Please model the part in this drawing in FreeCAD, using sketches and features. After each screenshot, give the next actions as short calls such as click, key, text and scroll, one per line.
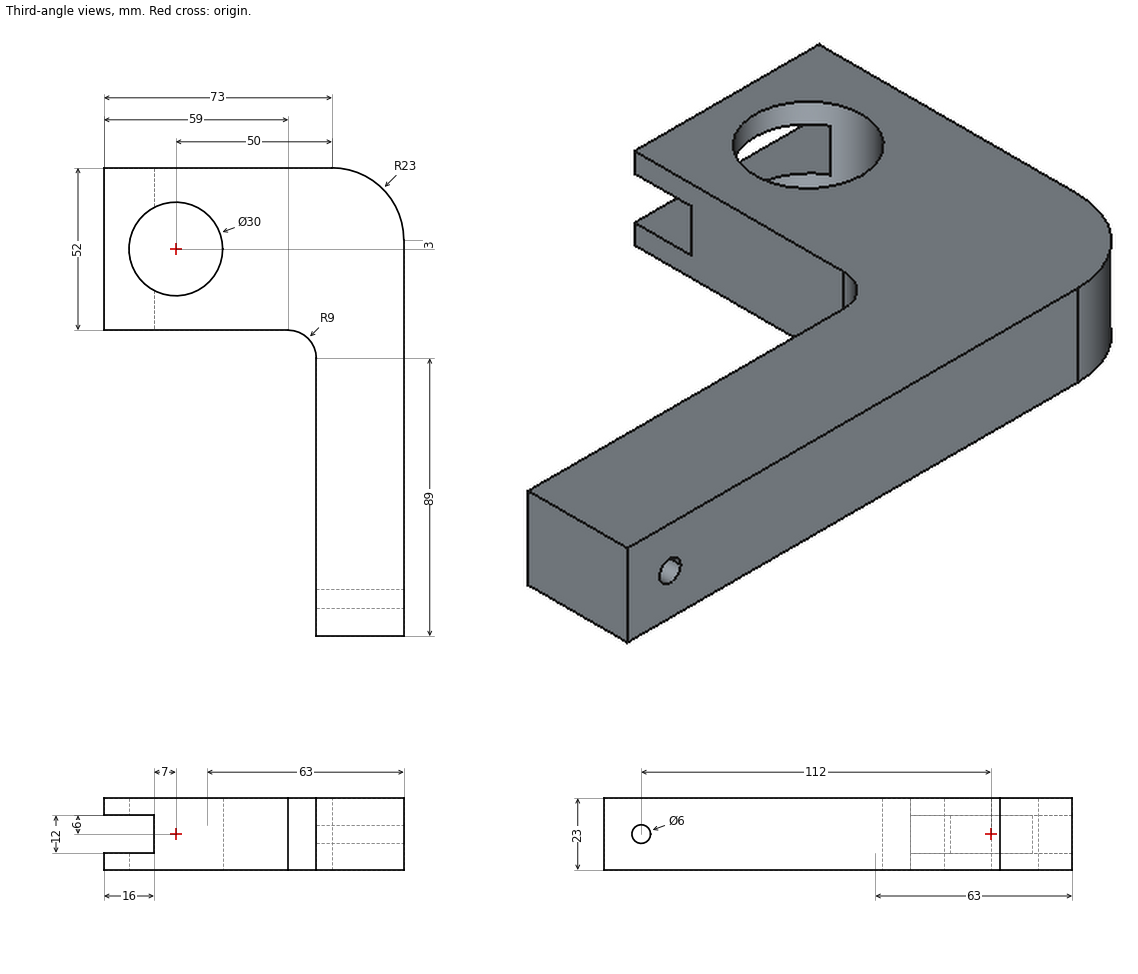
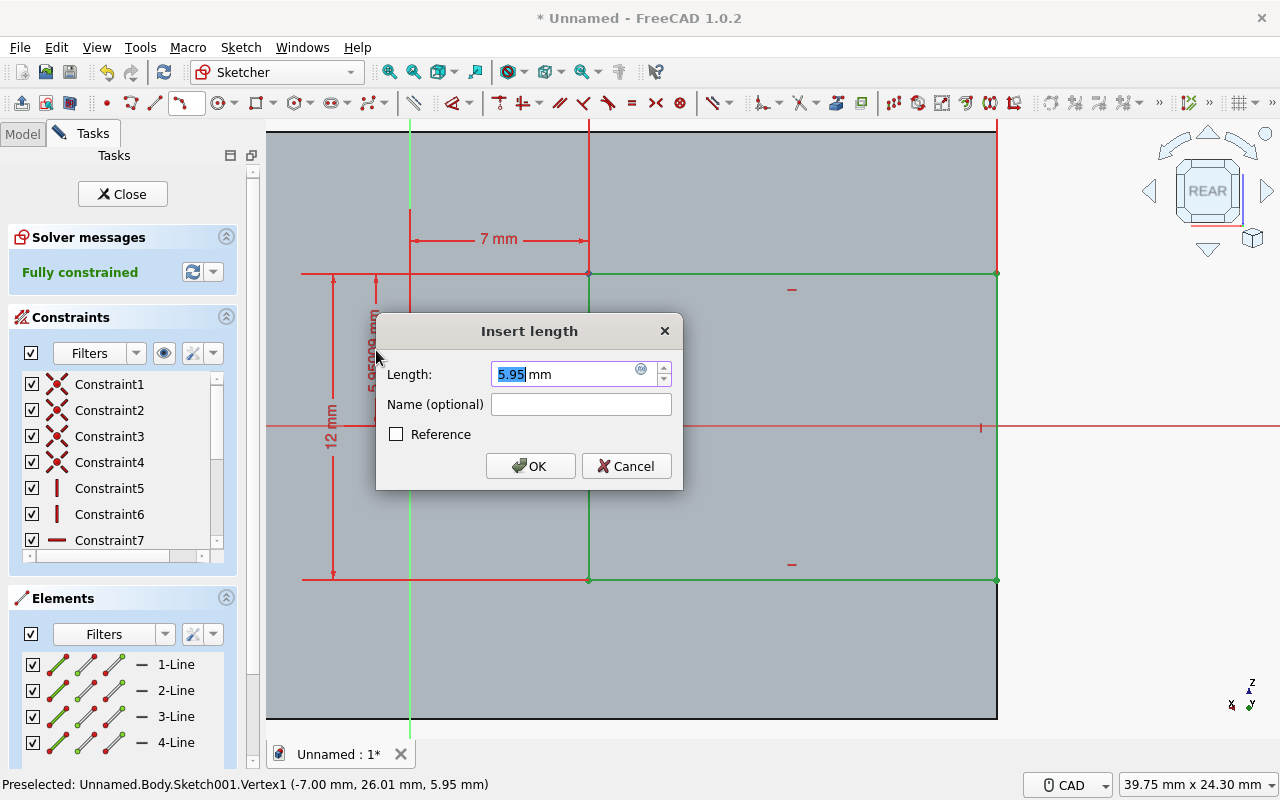
text(6)
key(Return)
key(Escape)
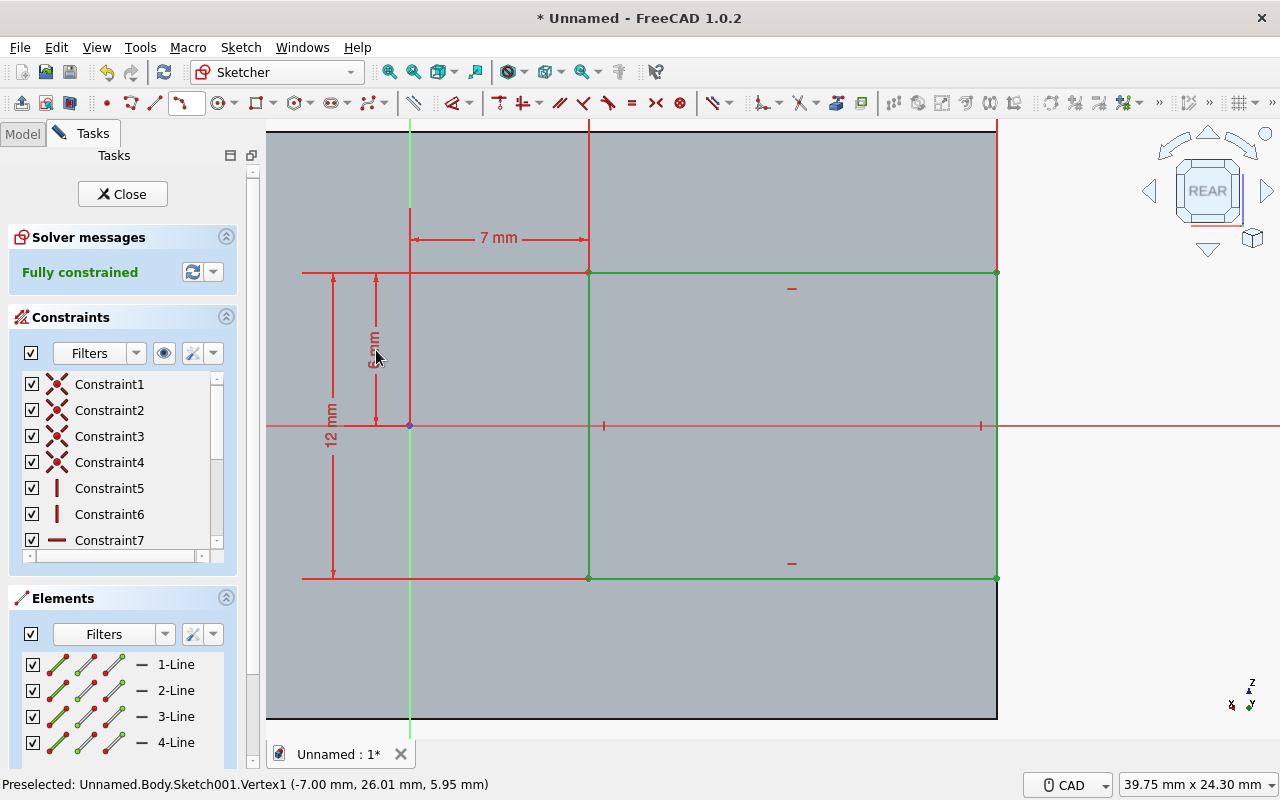
click(123, 194)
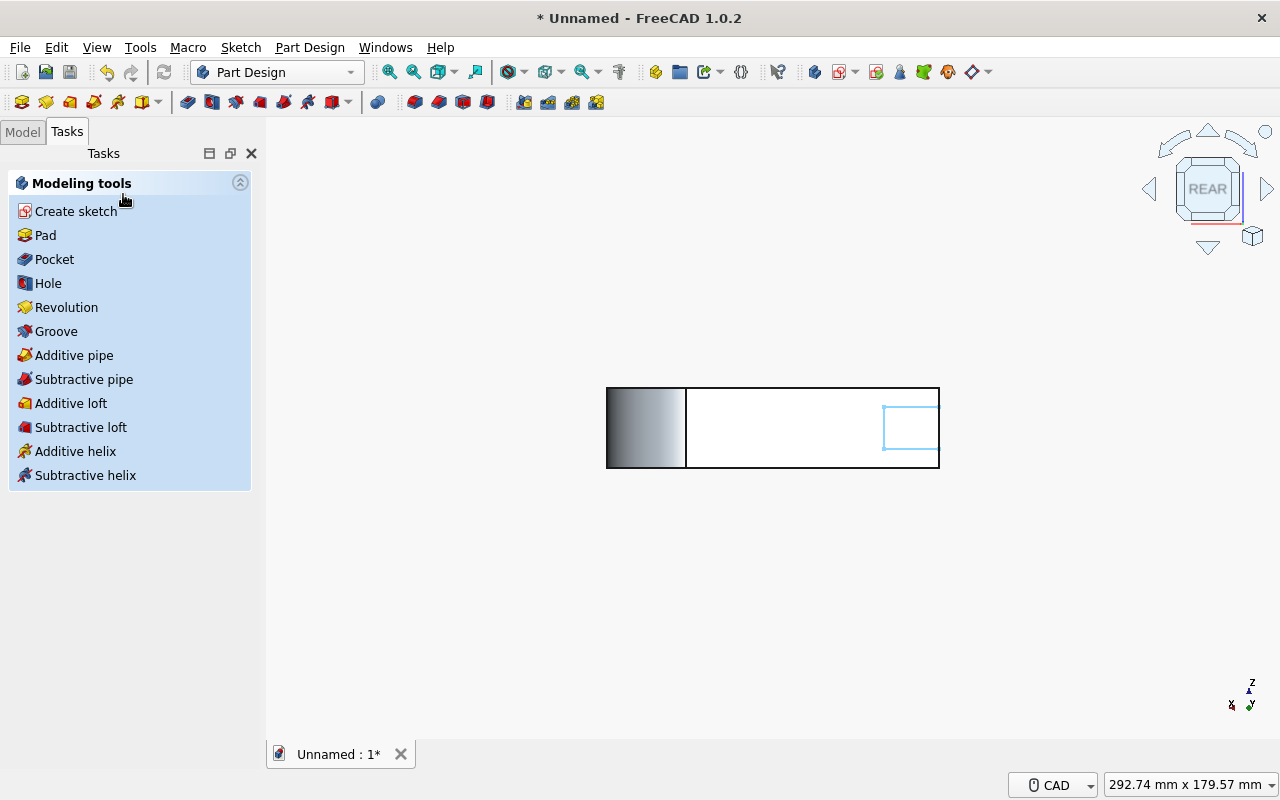
click(188, 102)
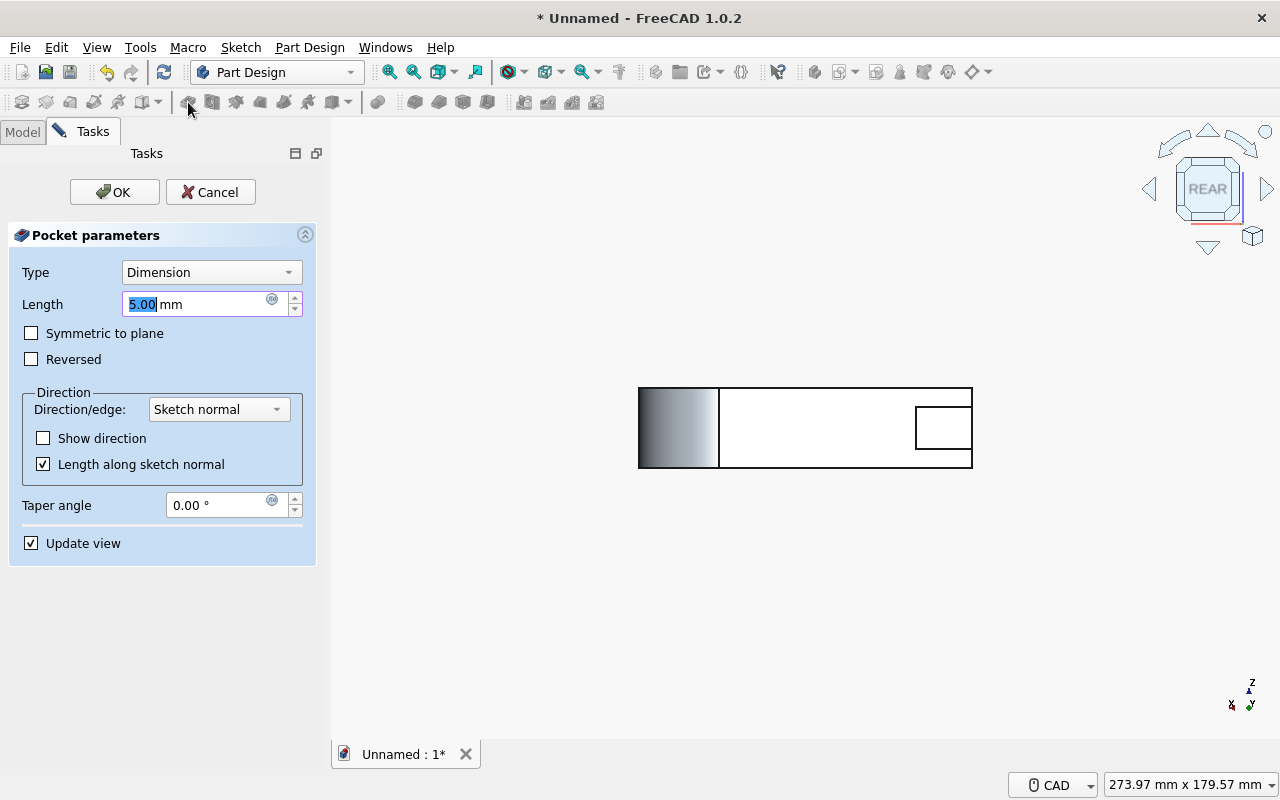
text(63)
key(Tab)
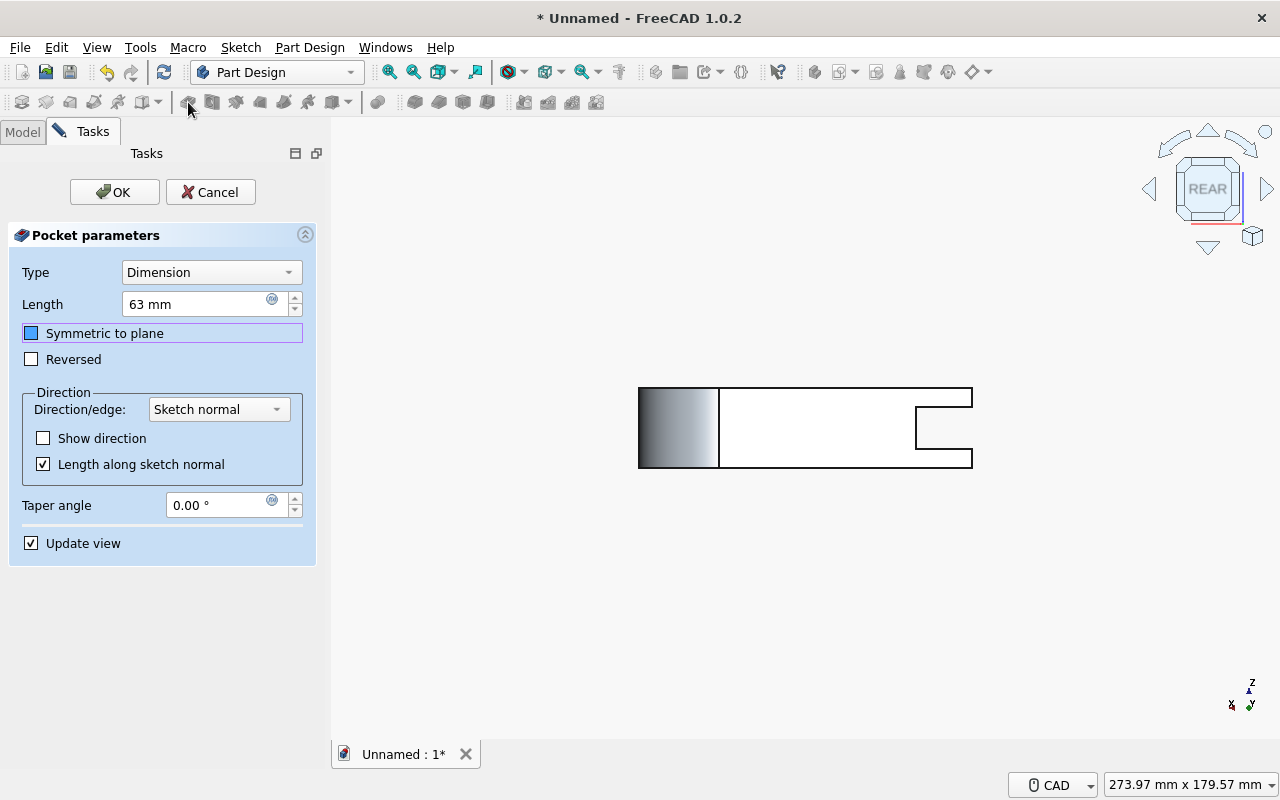
click(115, 192)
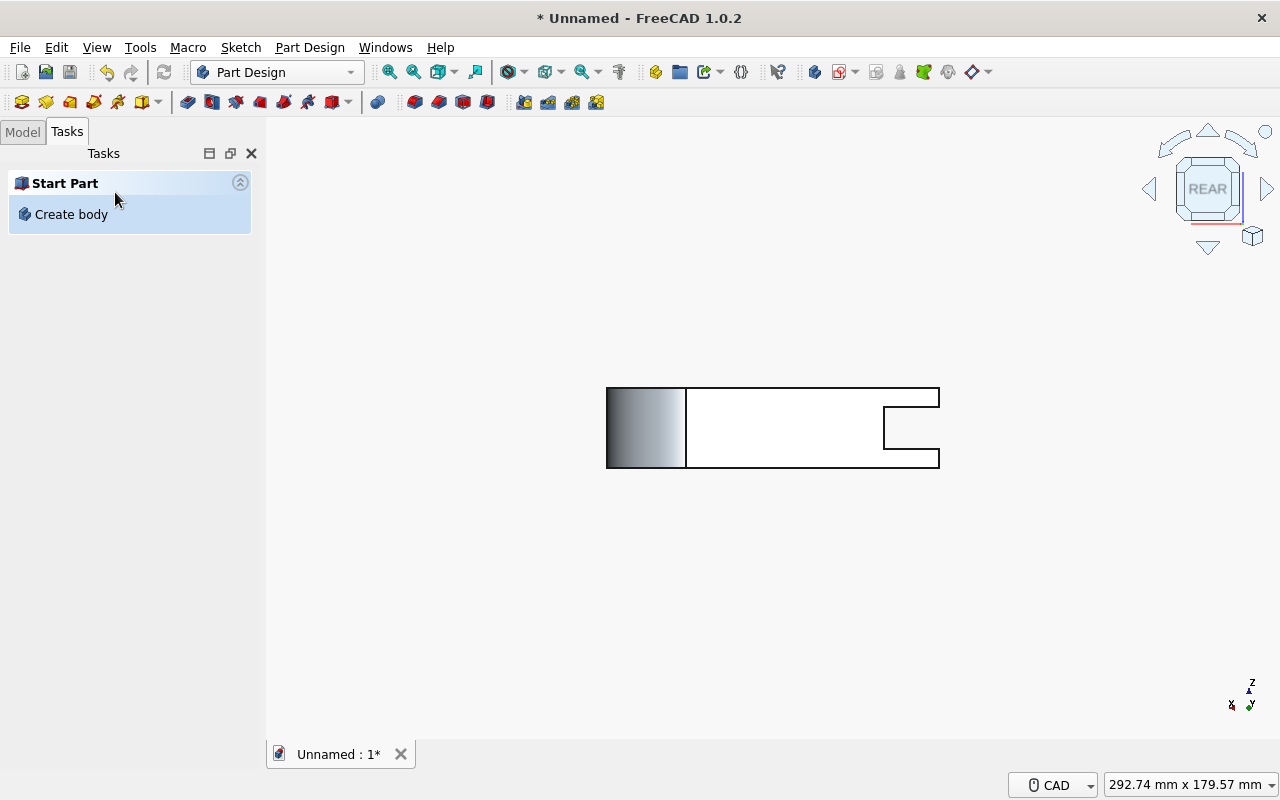
click(390, 72)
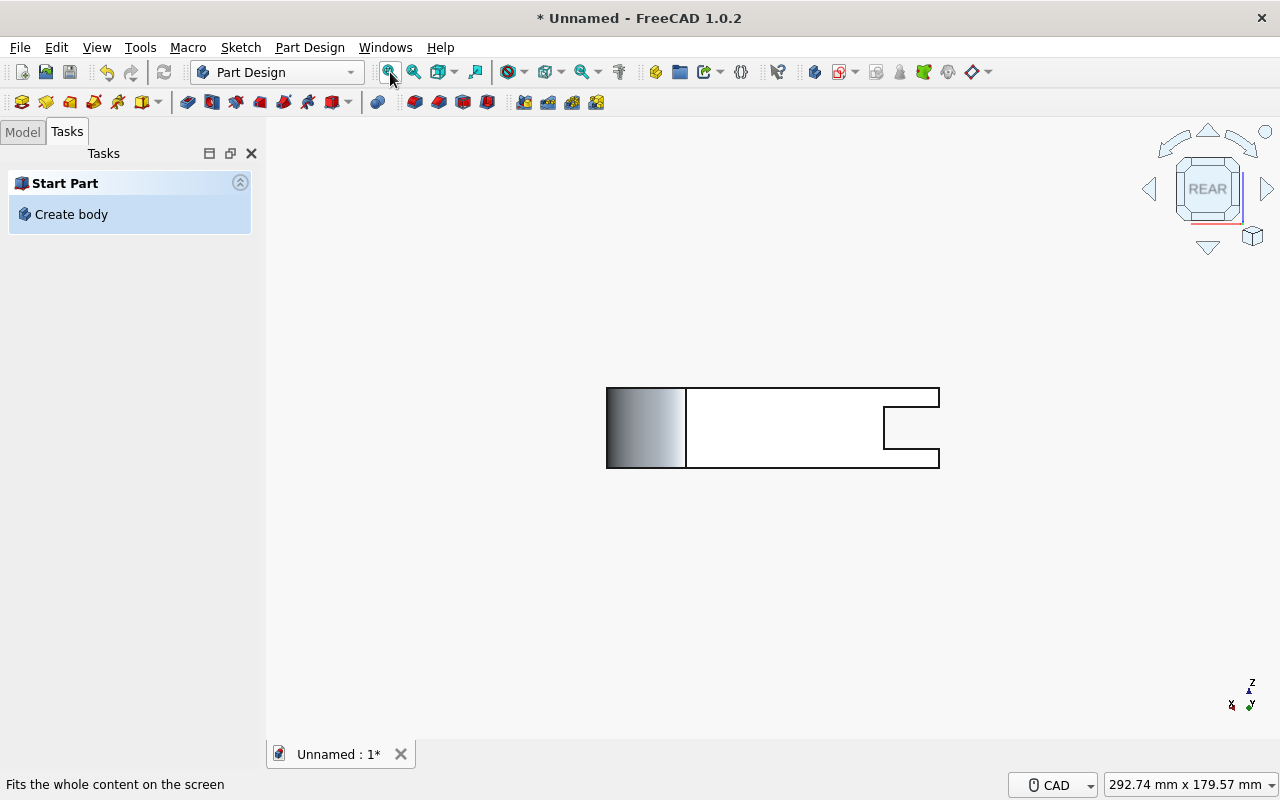
key(0)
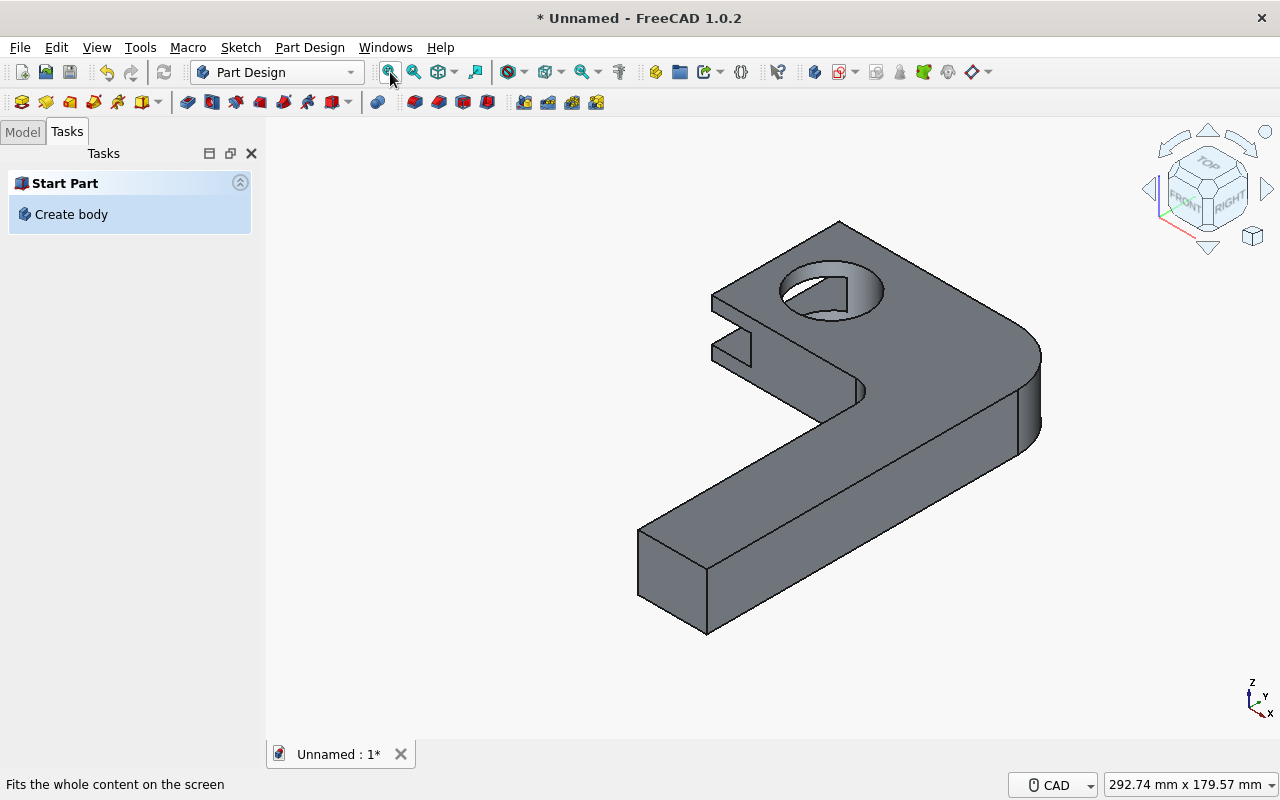
click(951, 460)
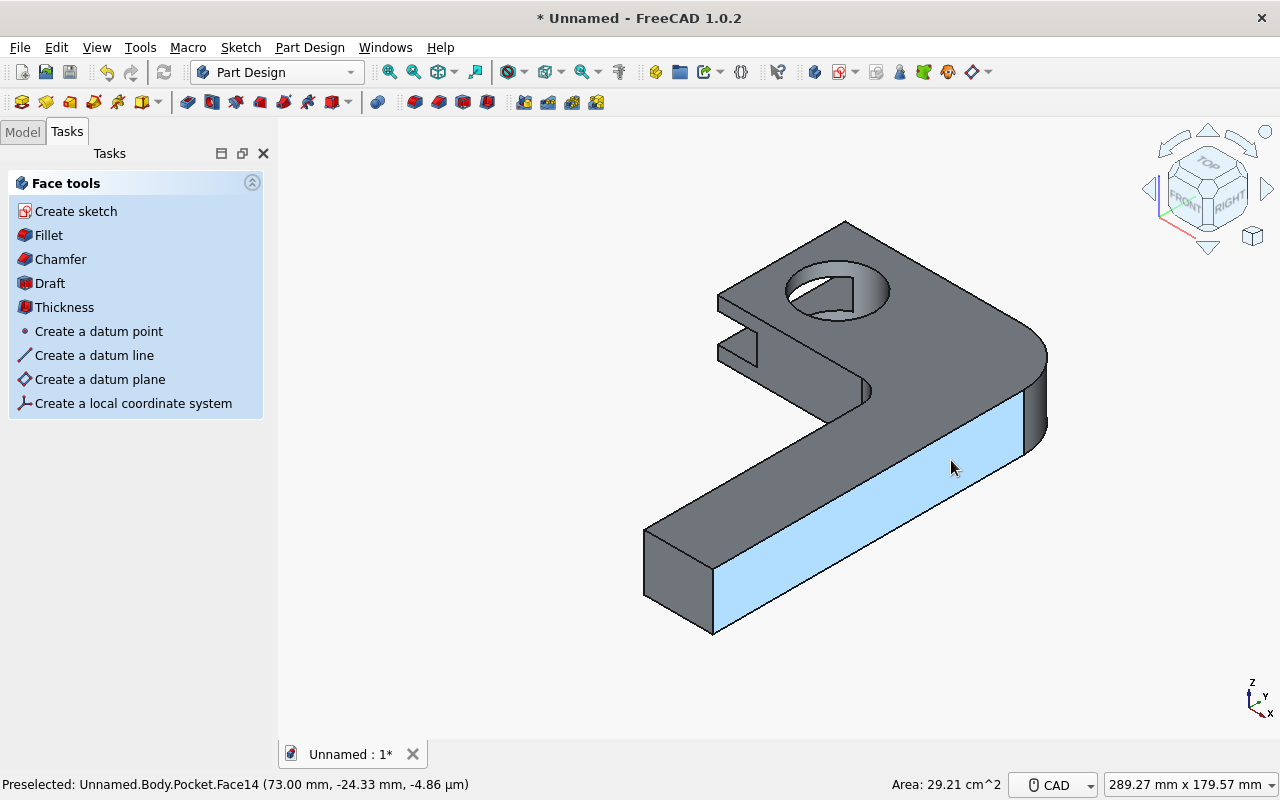
click(840, 72)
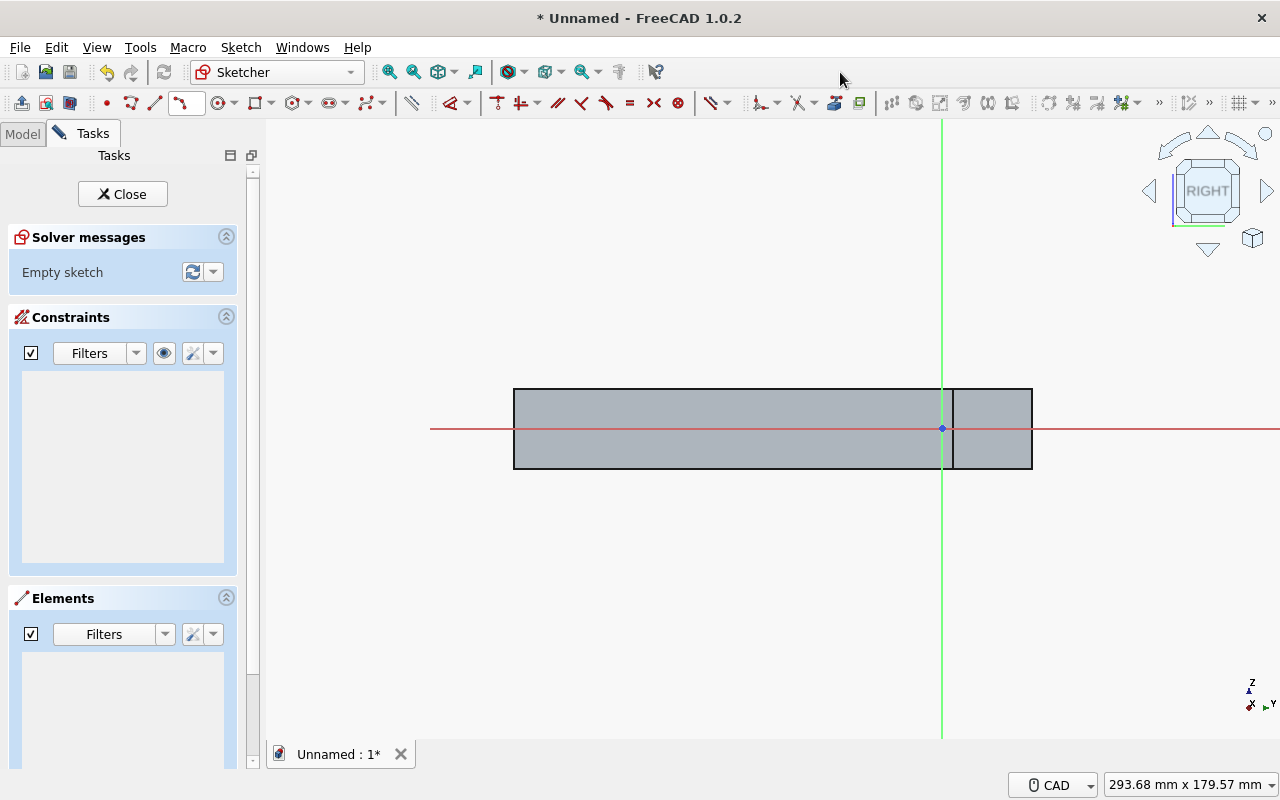
scroll(548, 429, up, 15)